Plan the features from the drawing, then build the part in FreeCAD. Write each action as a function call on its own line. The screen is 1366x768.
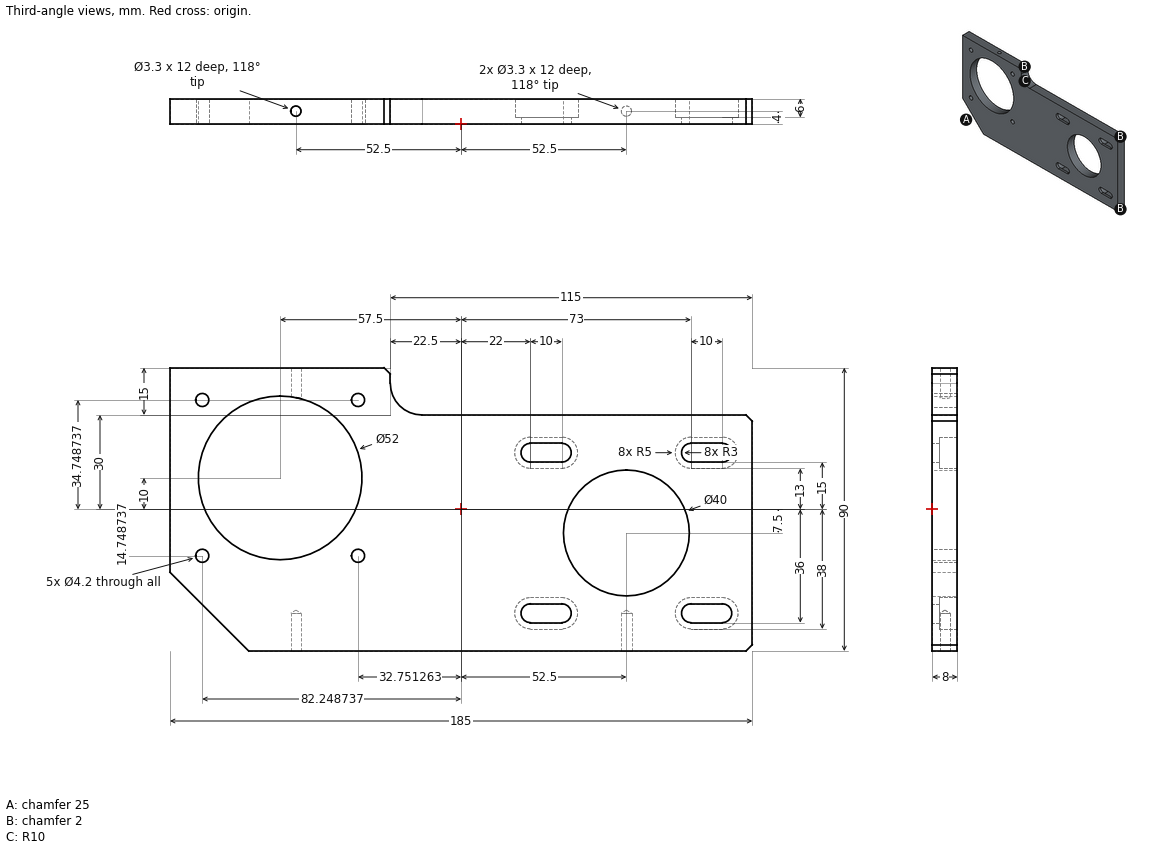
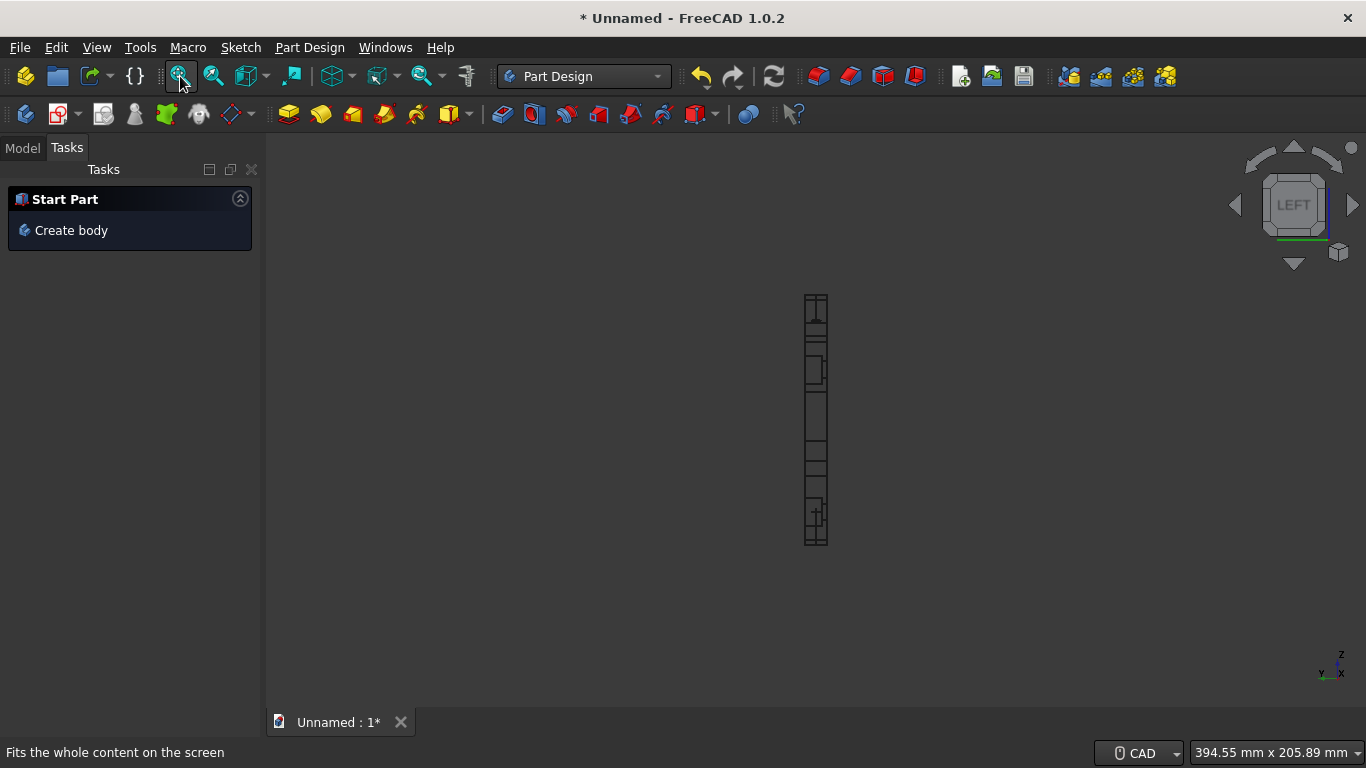
key(0)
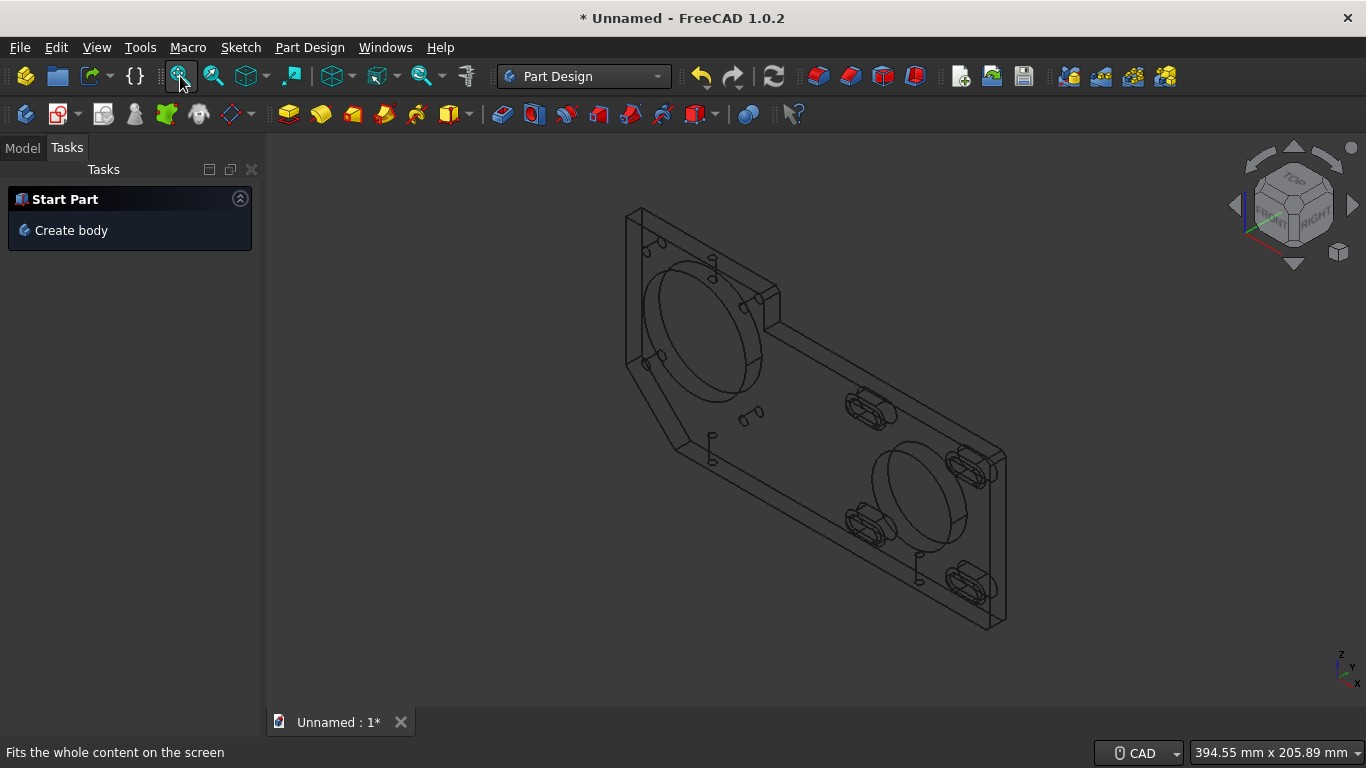
click(772, 325)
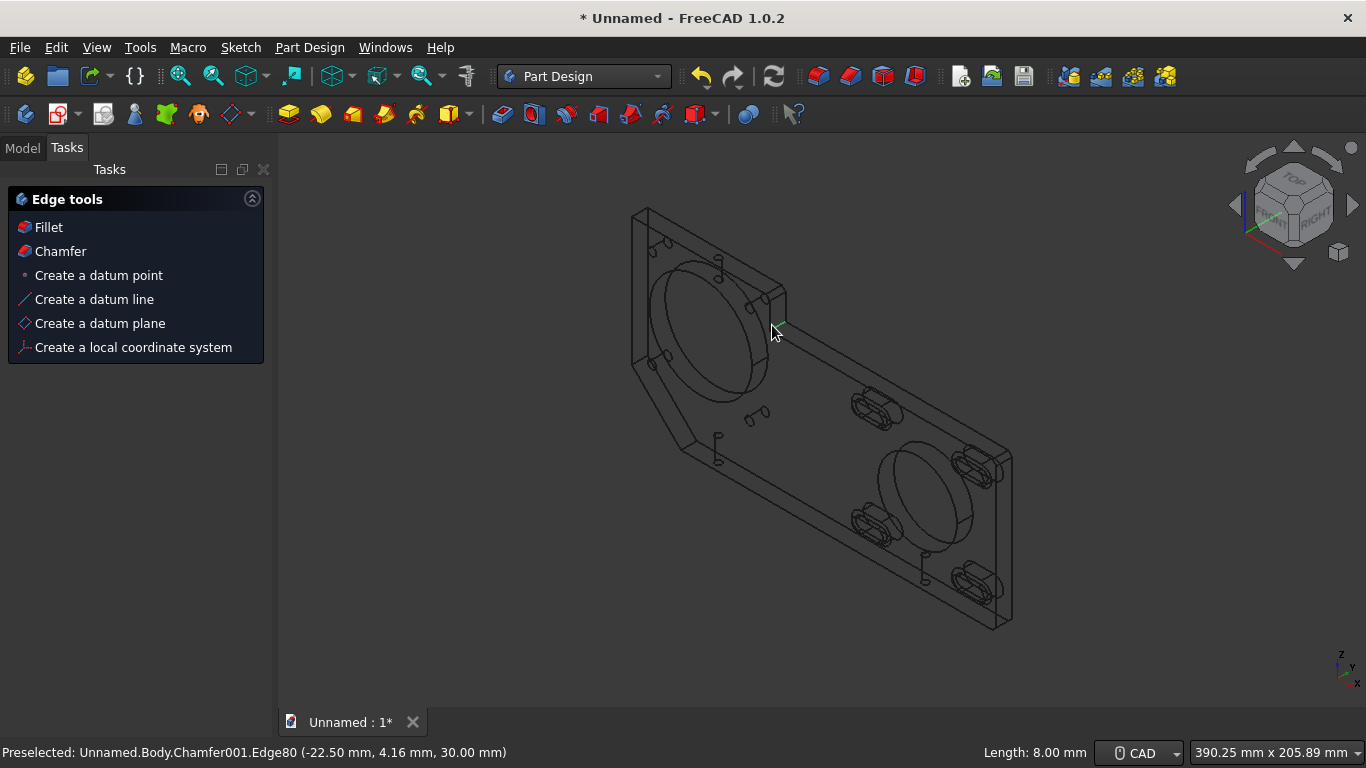
key(v)
key(1)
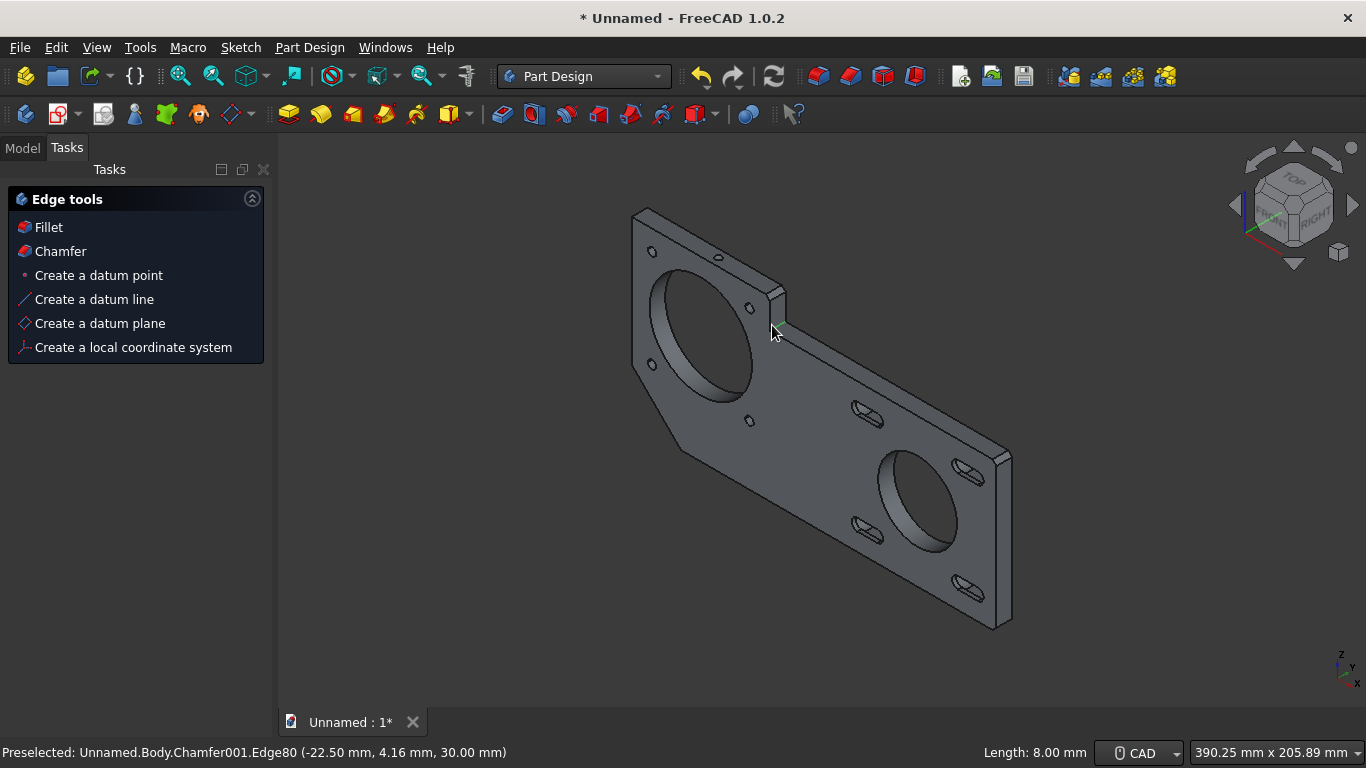
click(820, 76)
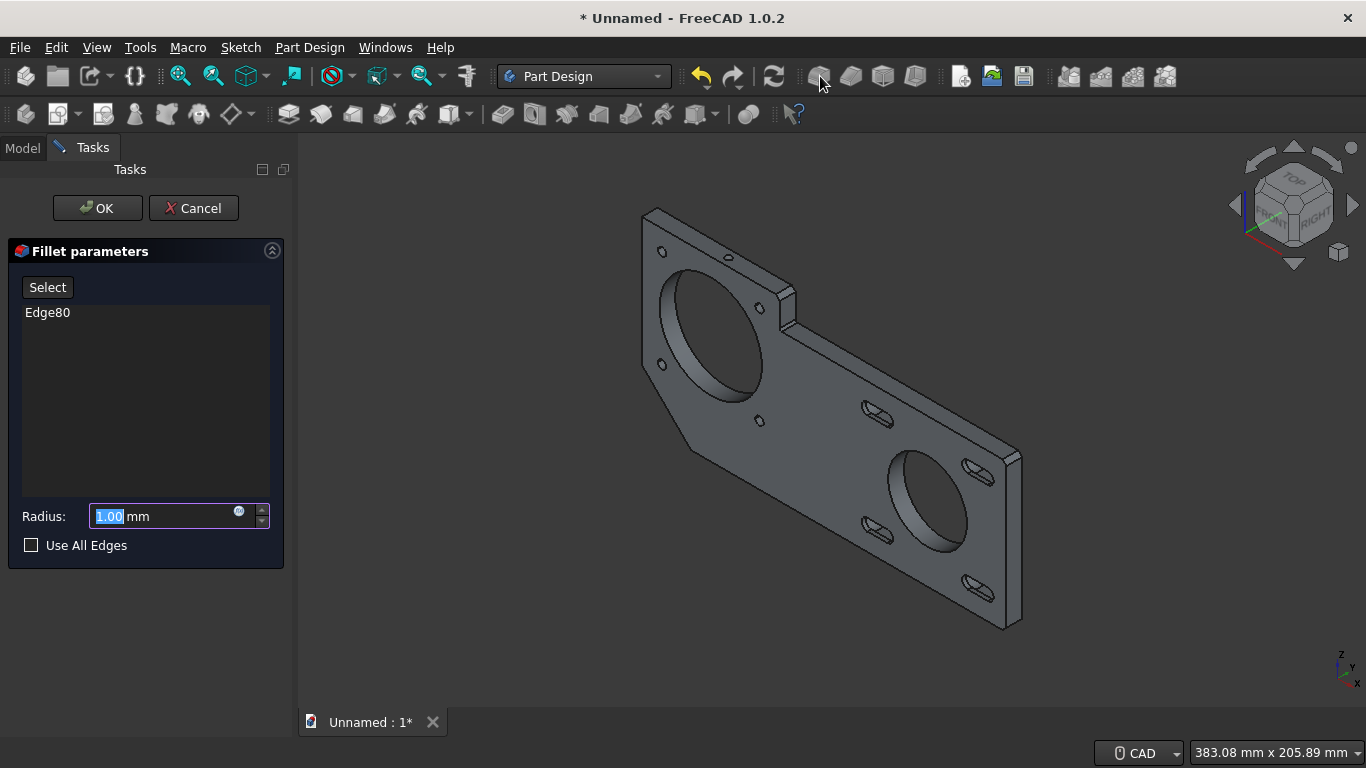
text(10)
key(Tab)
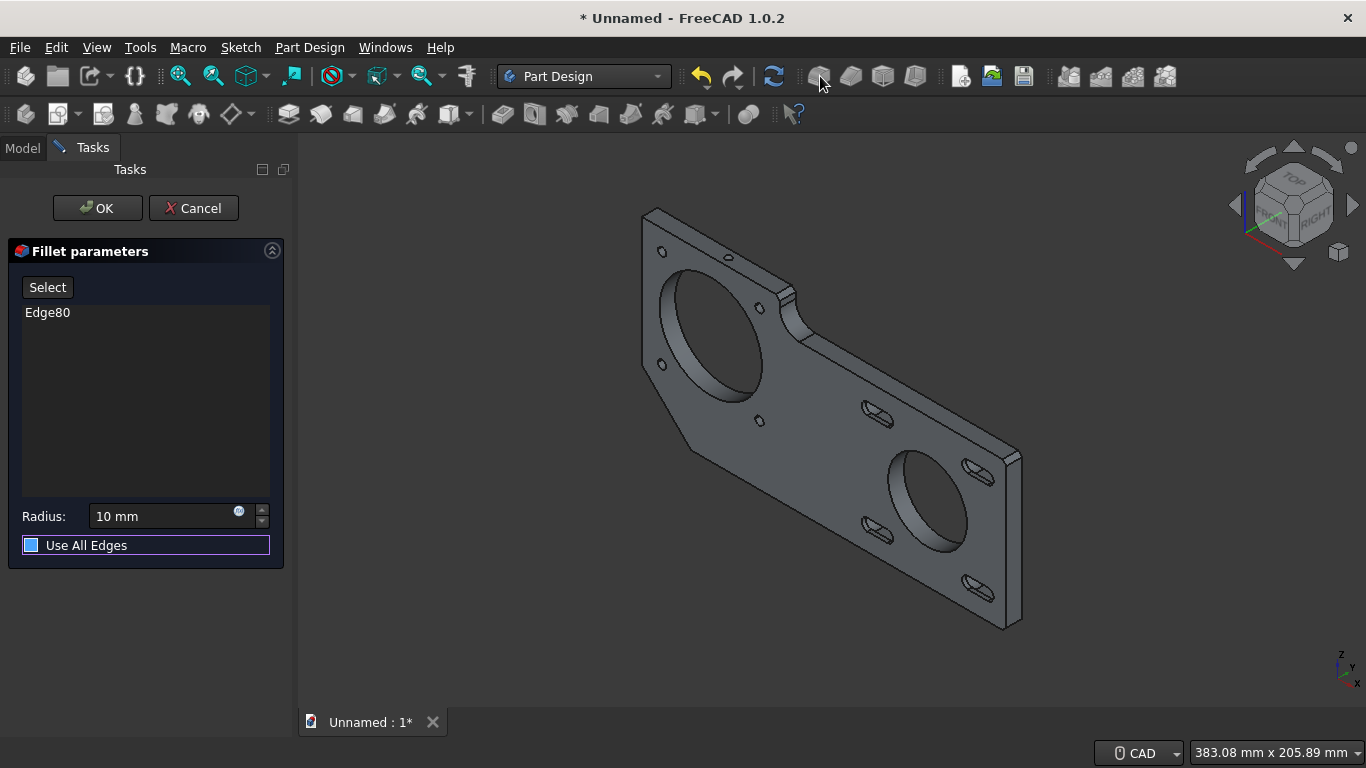
click(98, 208)